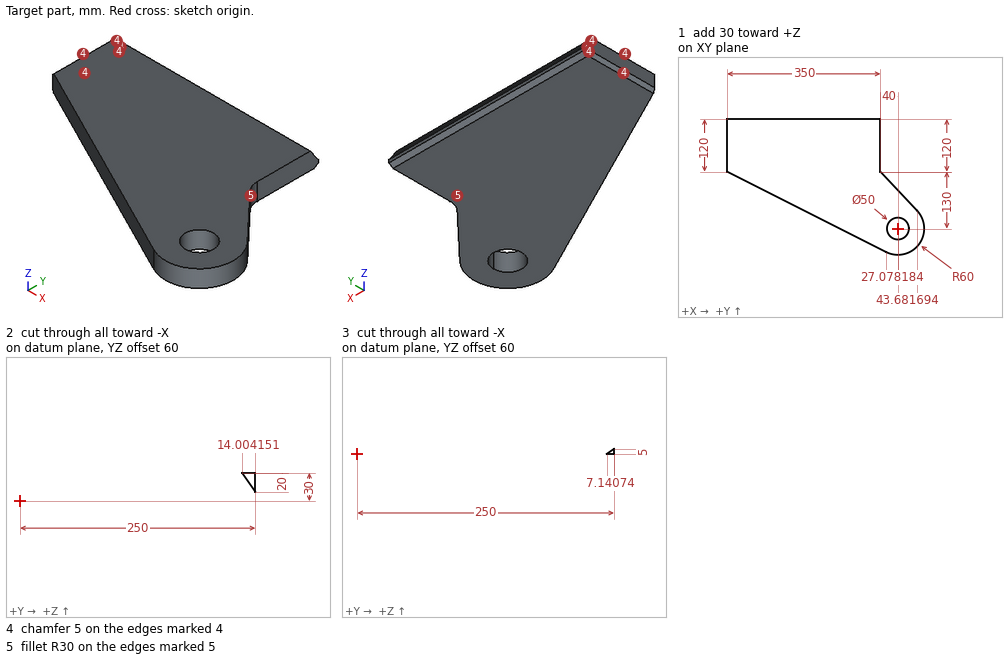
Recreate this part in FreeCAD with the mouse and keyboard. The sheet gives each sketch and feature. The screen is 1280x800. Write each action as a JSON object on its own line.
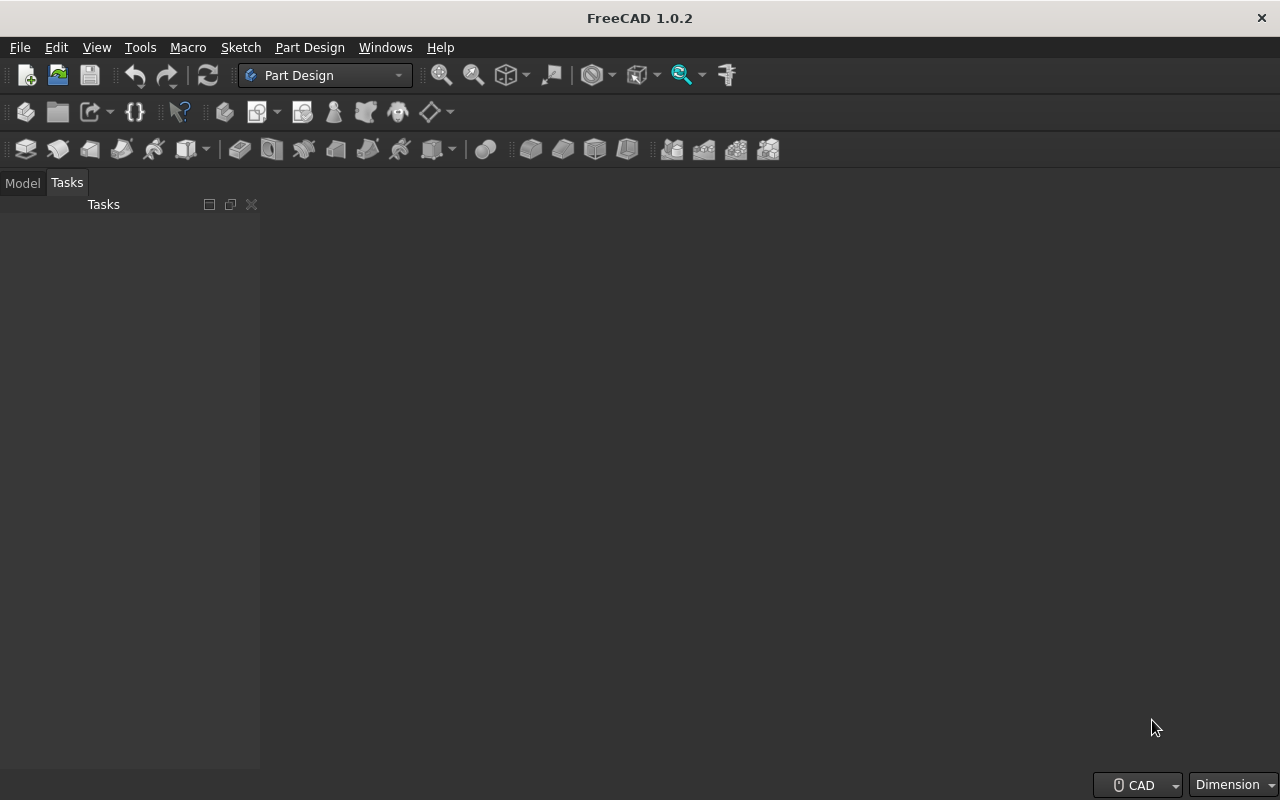
{"action": "key", "text": "ctrl+n"}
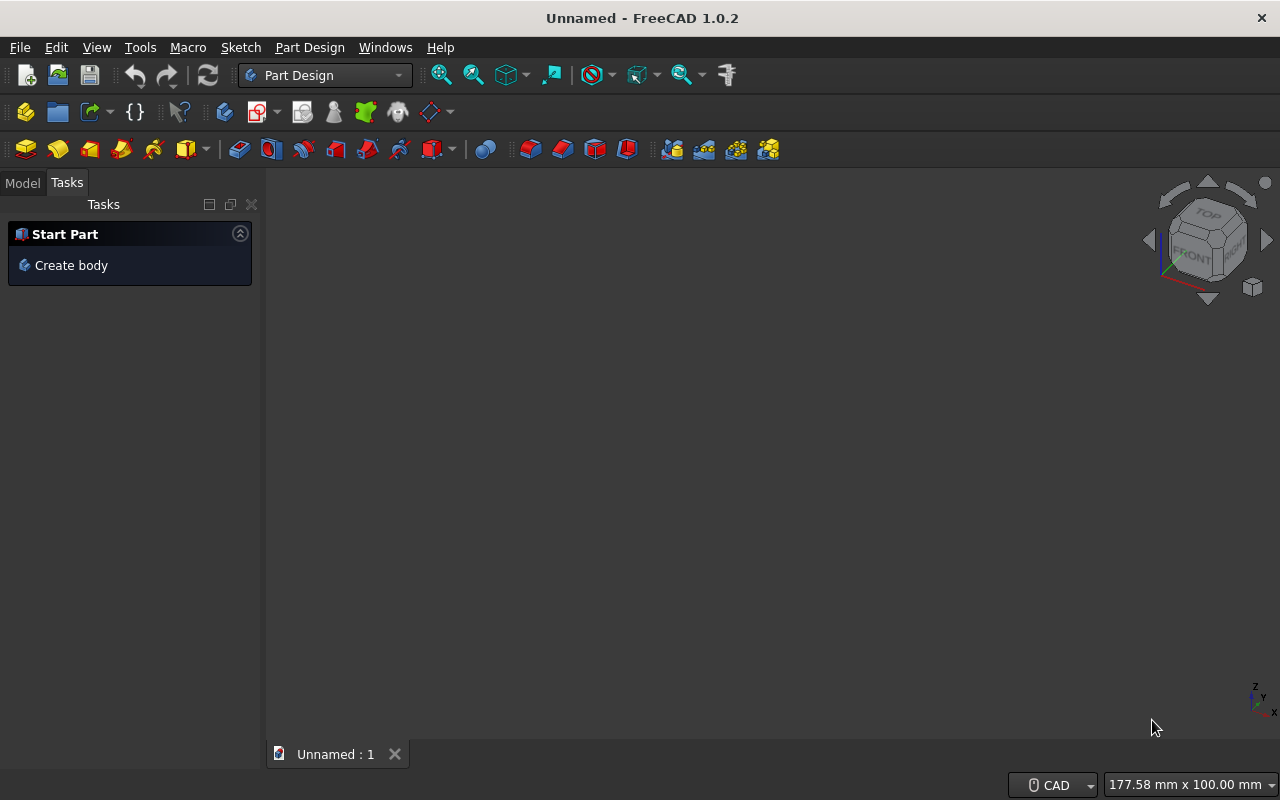
{"action": "left_click", "coordinate": [258, 112]}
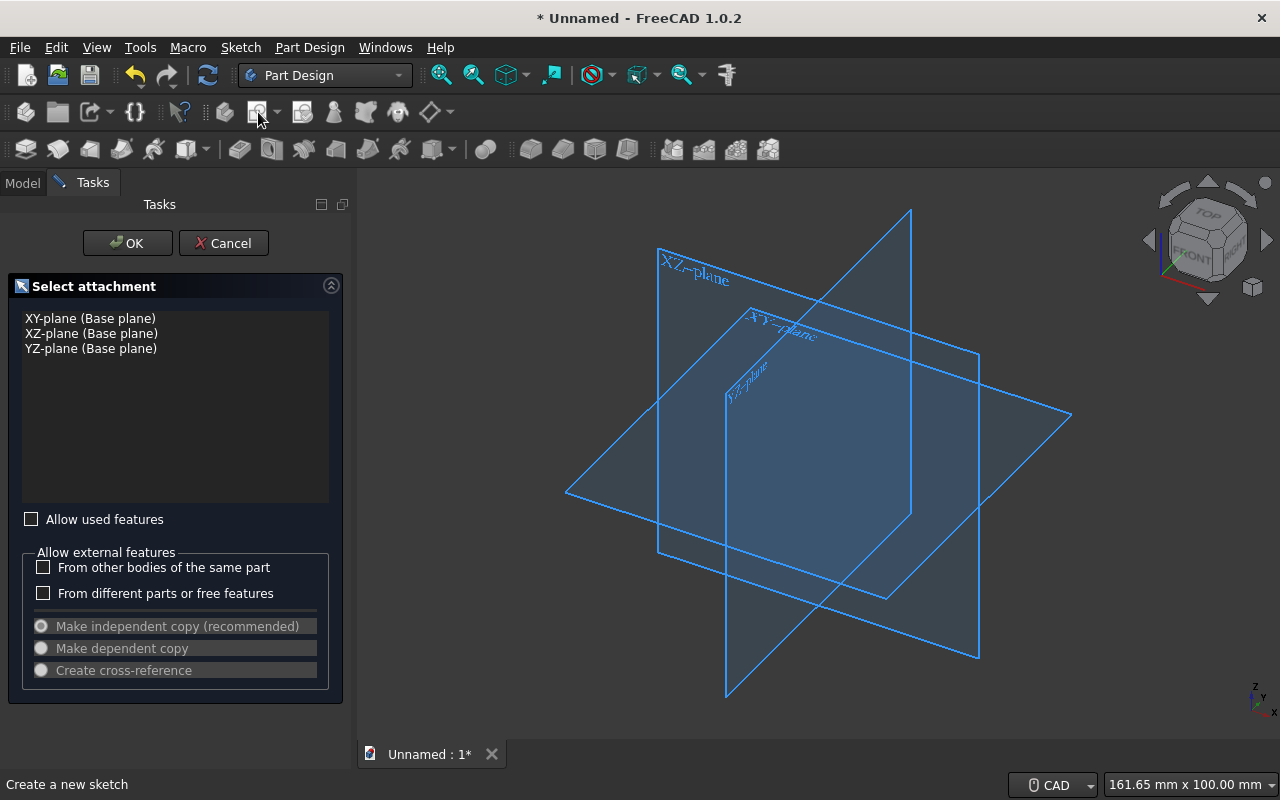
{"action": "left_click", "coordinate": [82, 318]}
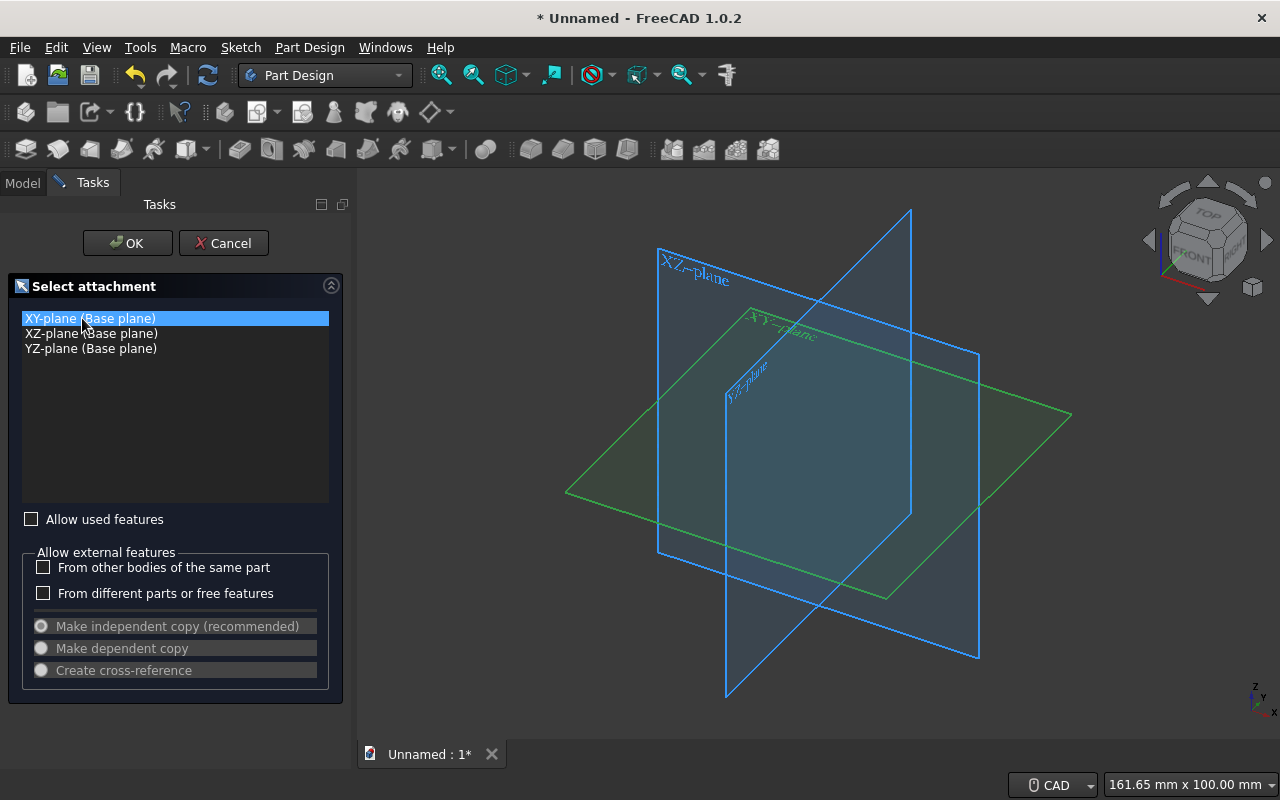
{"action": "left_click", "coordinate": [128, 243]}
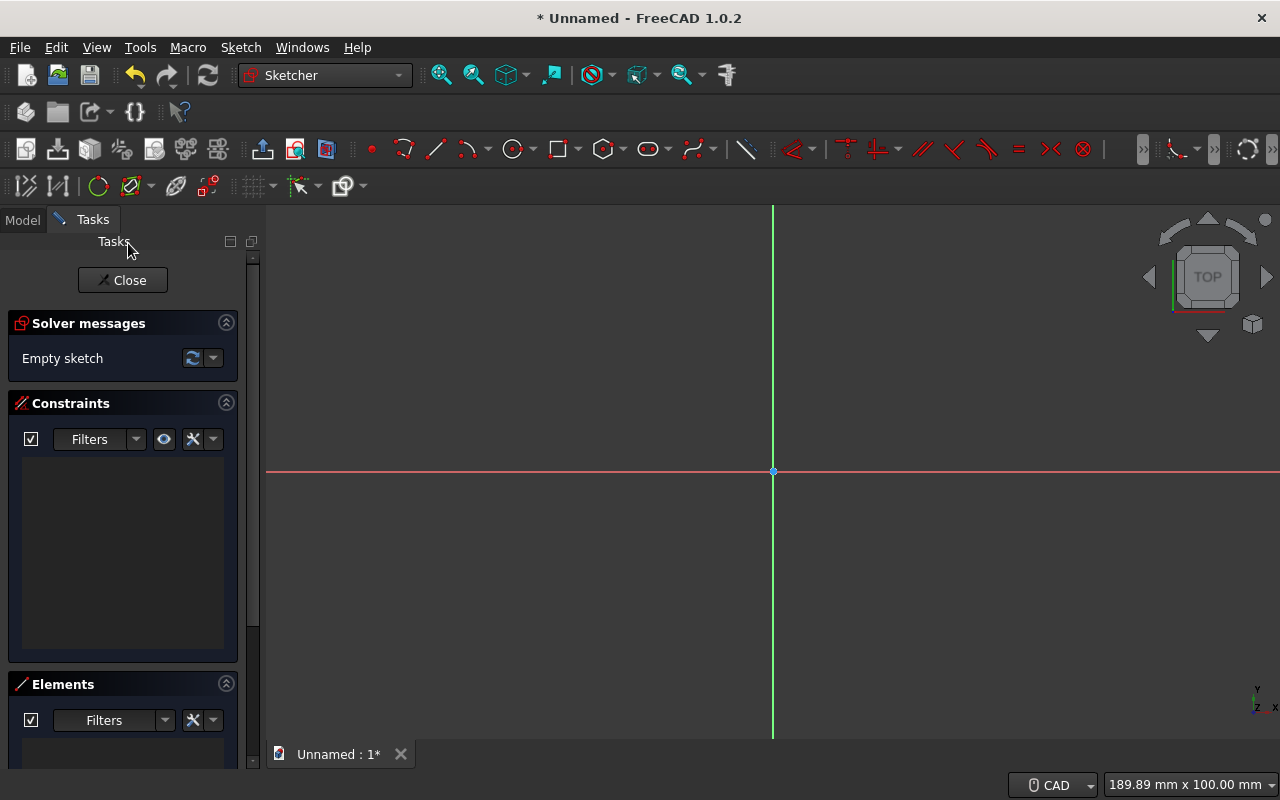
{"action": "scroll", "coordinate": [918, 605], "scroll_direction": "down", "scroll_amount": 8}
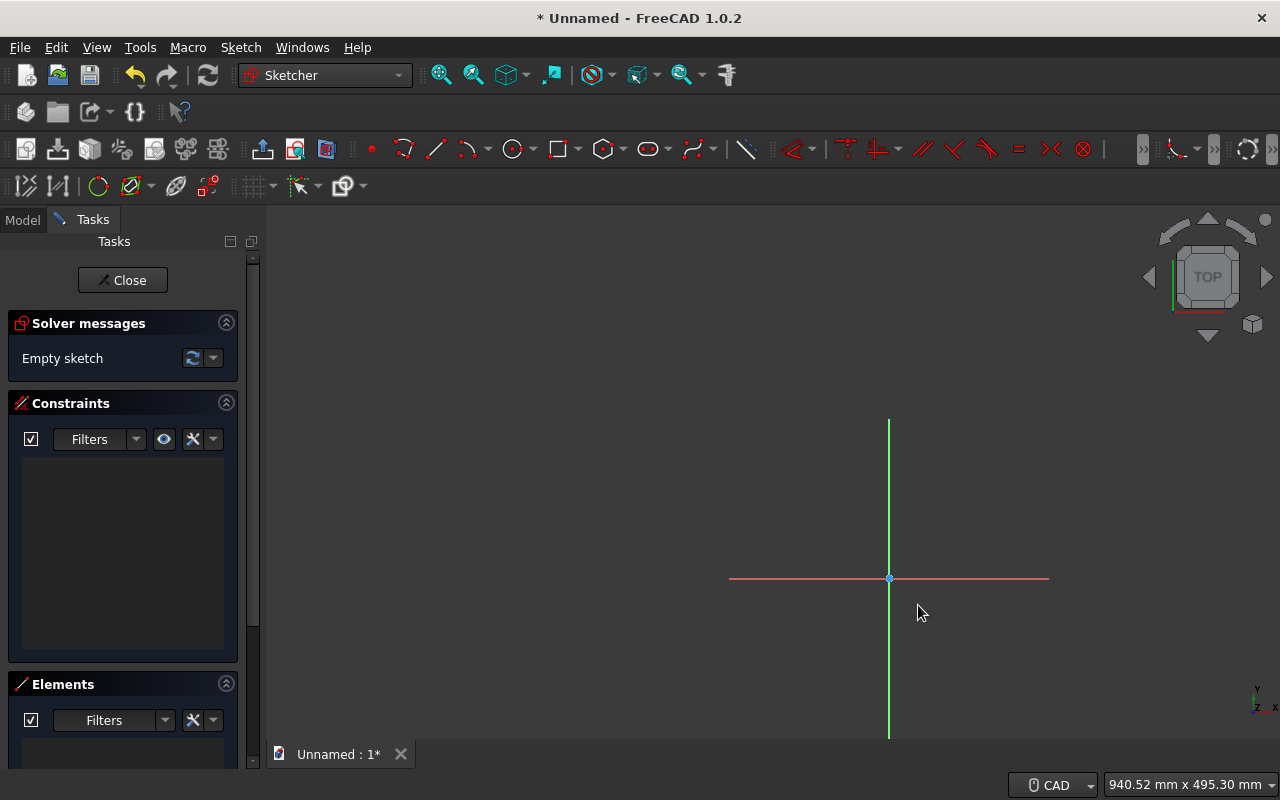
{"action": "key", "text": "g m"}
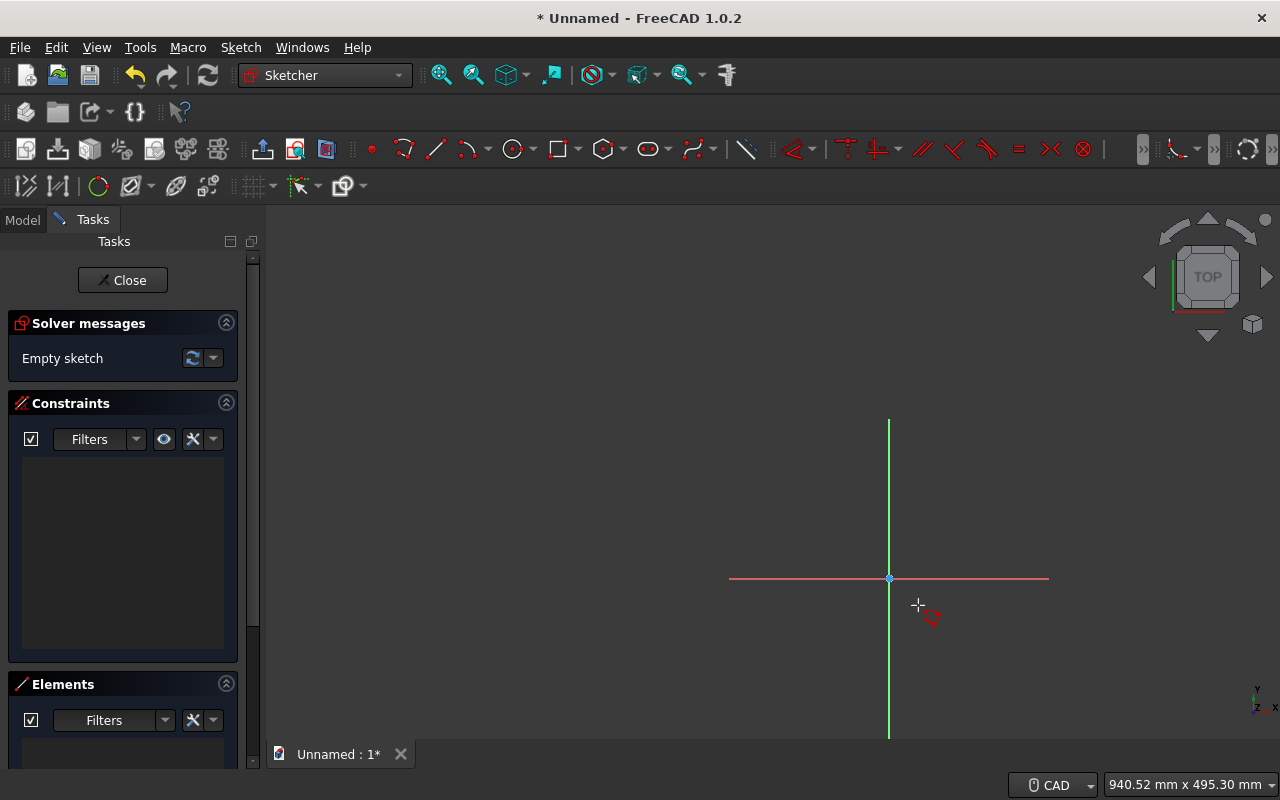
{"action": "left_click", "coordinate": [936, 534]}
{"action": "left_click", "coordinate": [846, 439]}
{"action": "left_click", "coordinate": [846, 309]}
{"action": "left_click", "coordinate": [469, 309]}
{"action": "left_click", "coordinate": [469, 439]}
{"action": "left_click", "coordinate": [860, 636]}
{"action": "right_click", "coordinate": [860, 636]}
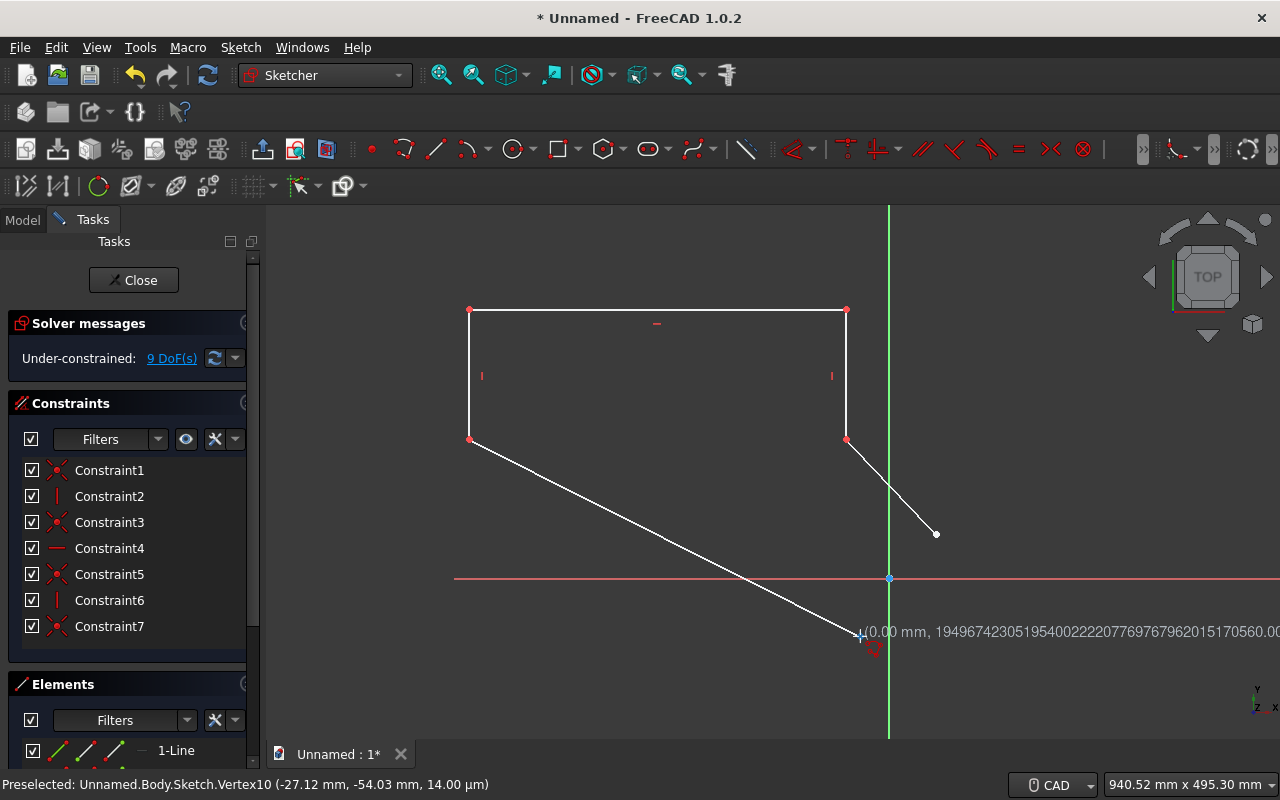
{"action": "key", "text": "g 3 a"}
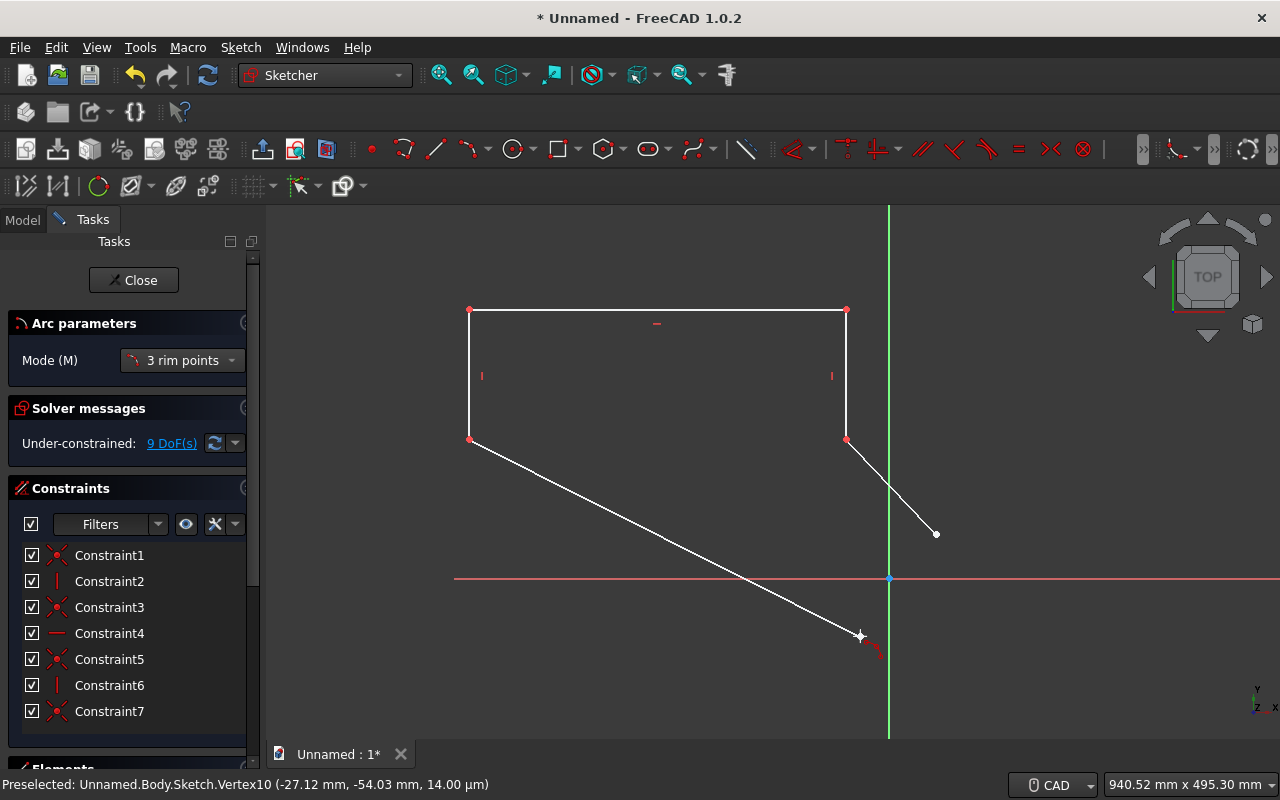
{"action": "left_click", "coordinate": [860, 637]}
{"action": "left_click", "coordinate": [936, 535]}
{"action": "left_click", "coordinate": [941, 617]}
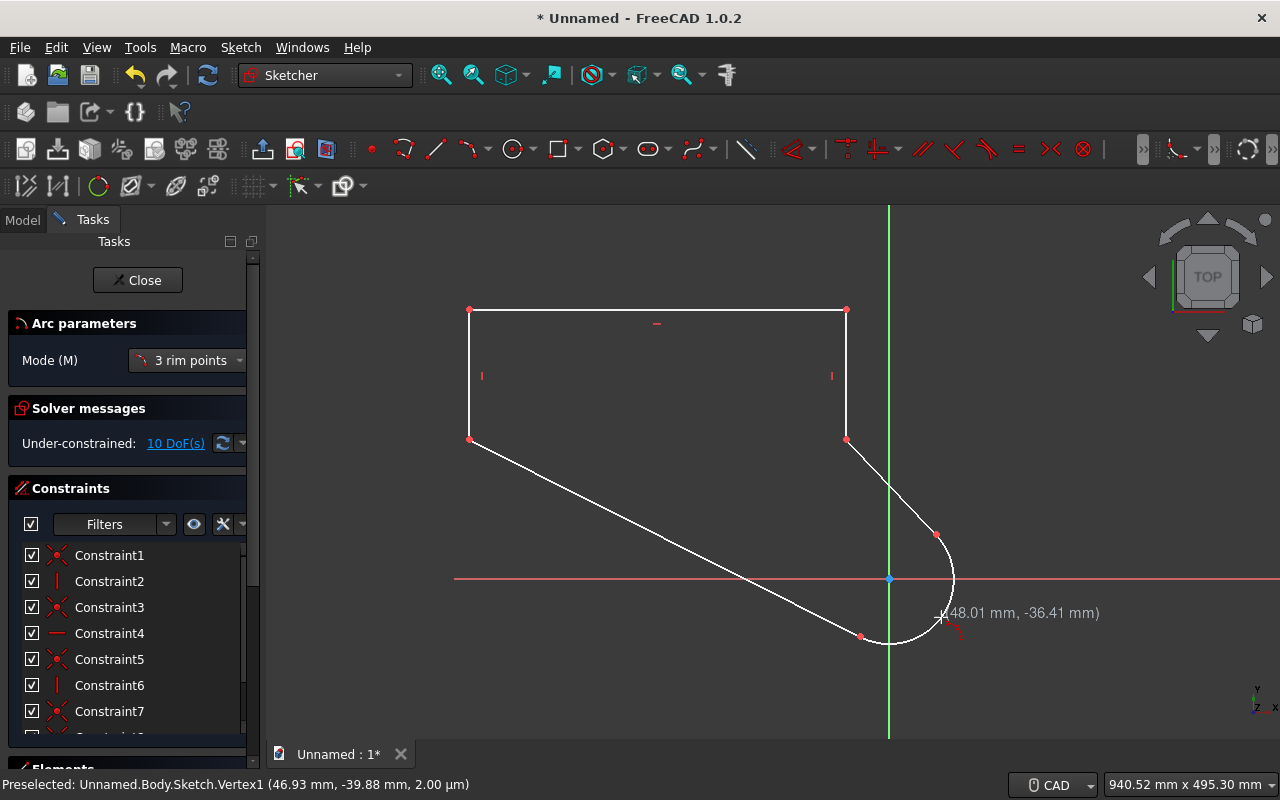
{"action": "left_click", "coordinate": [514, 150]}